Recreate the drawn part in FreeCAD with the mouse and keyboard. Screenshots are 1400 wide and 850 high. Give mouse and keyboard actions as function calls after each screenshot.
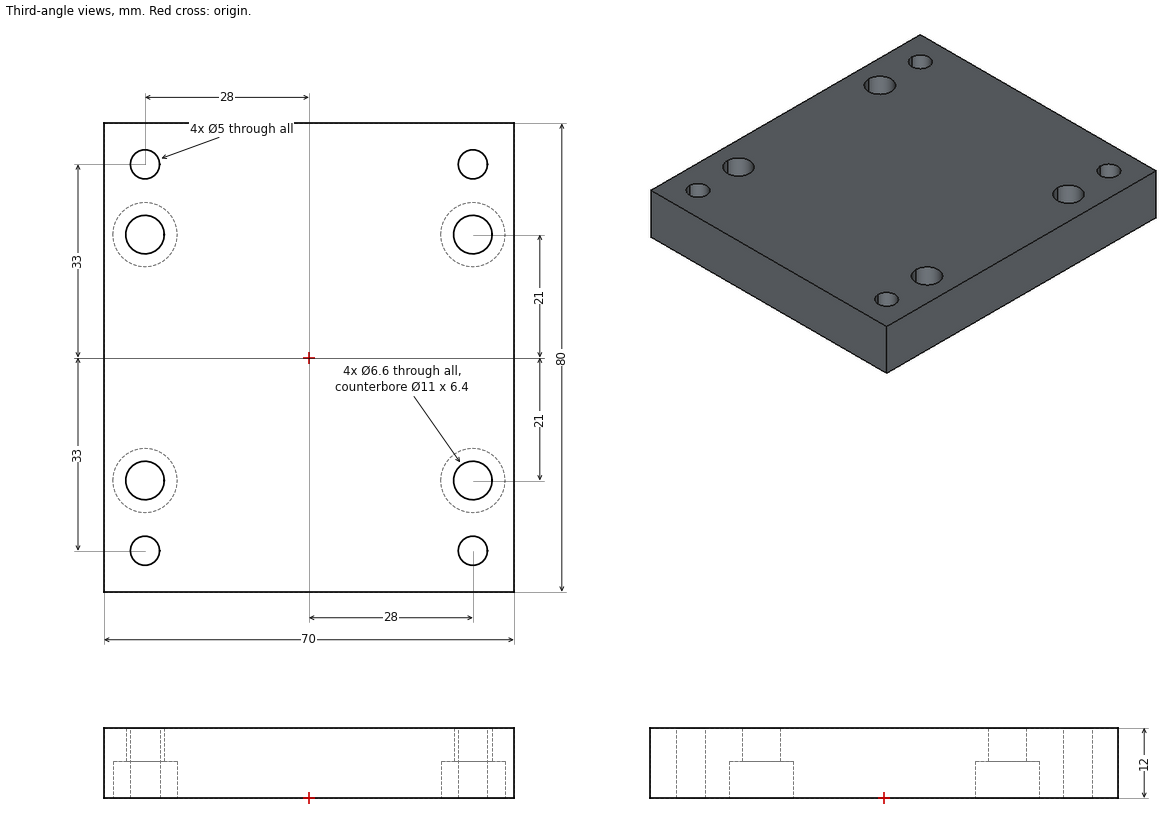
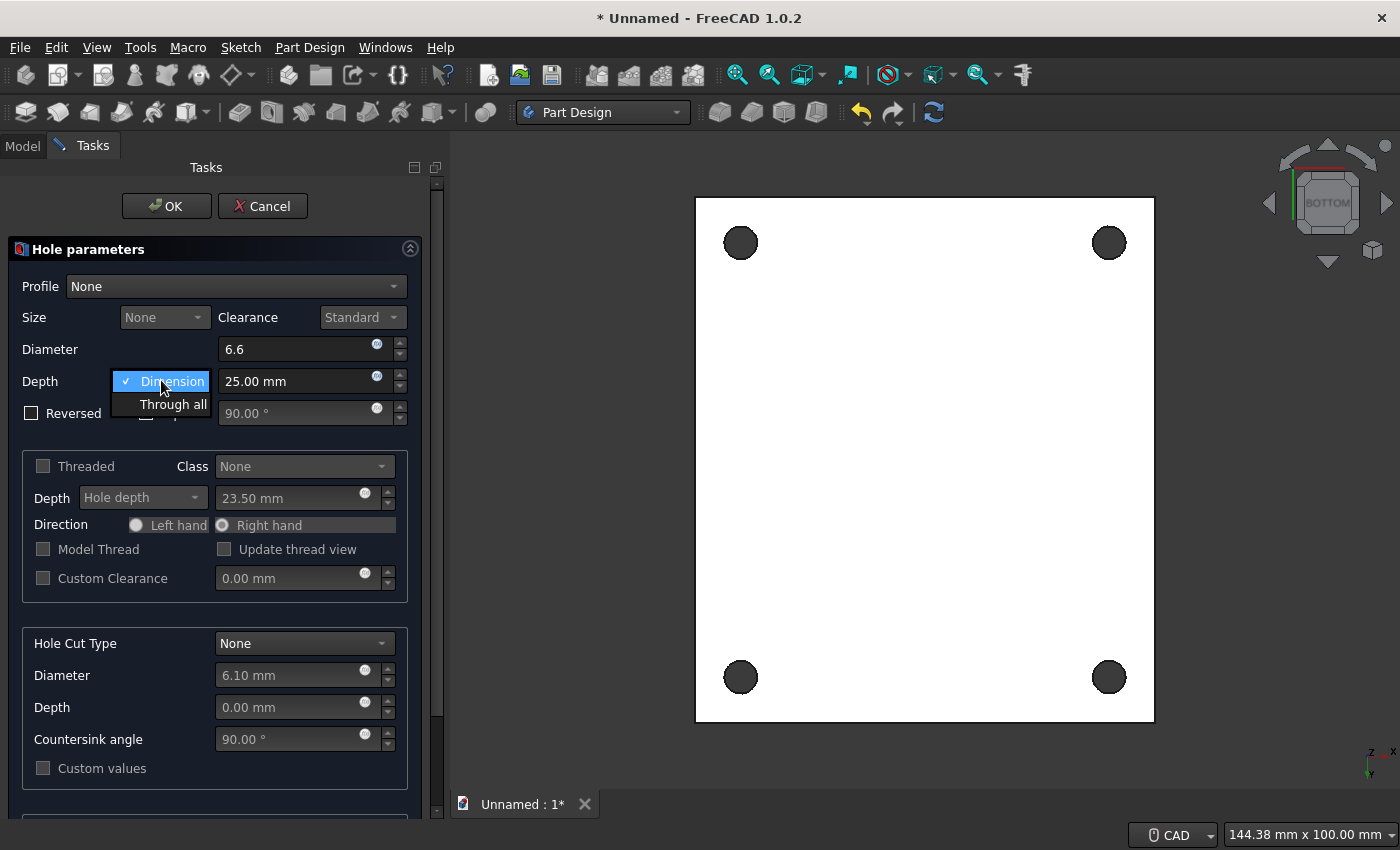
click(160, 404)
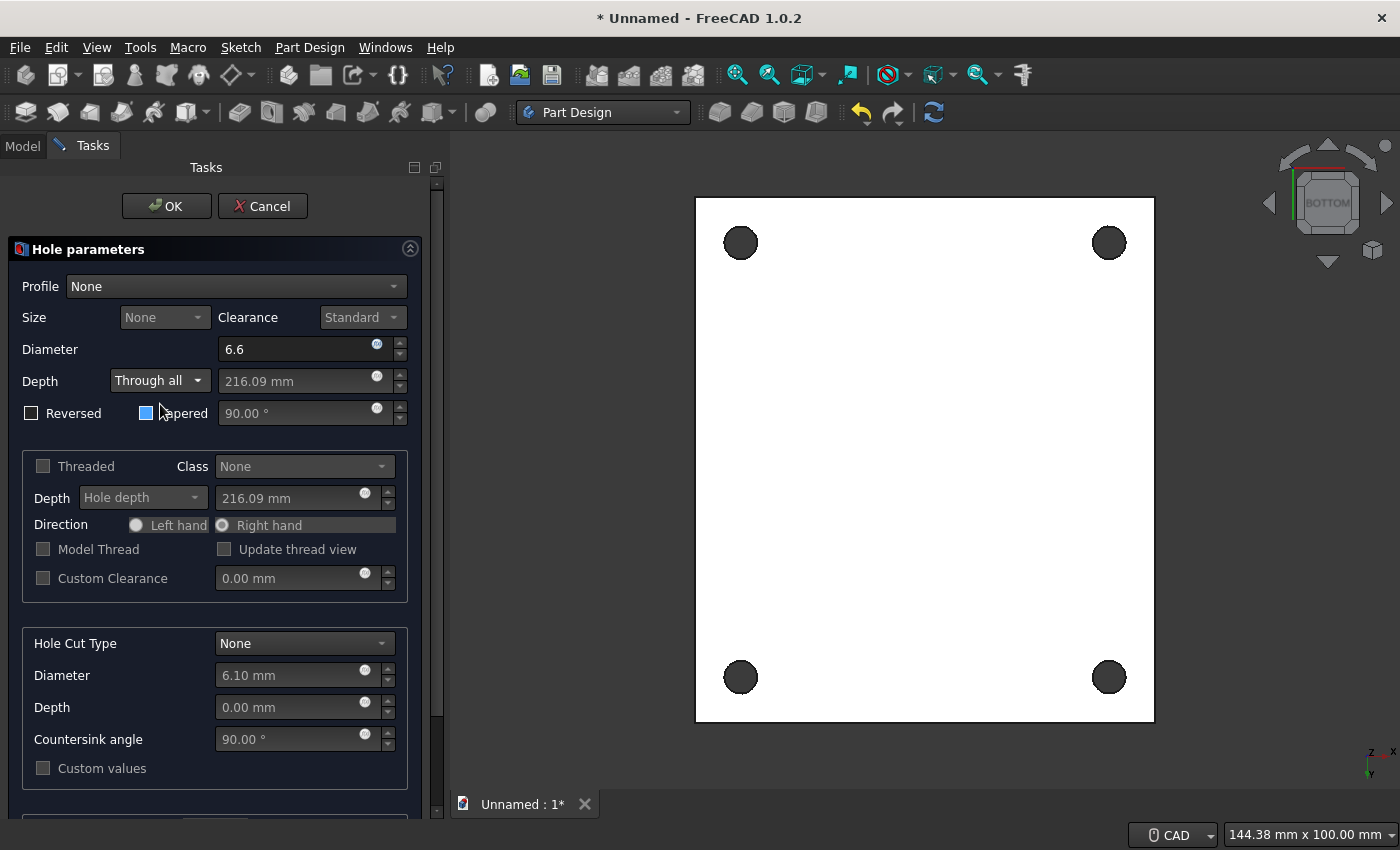
click(30, 413)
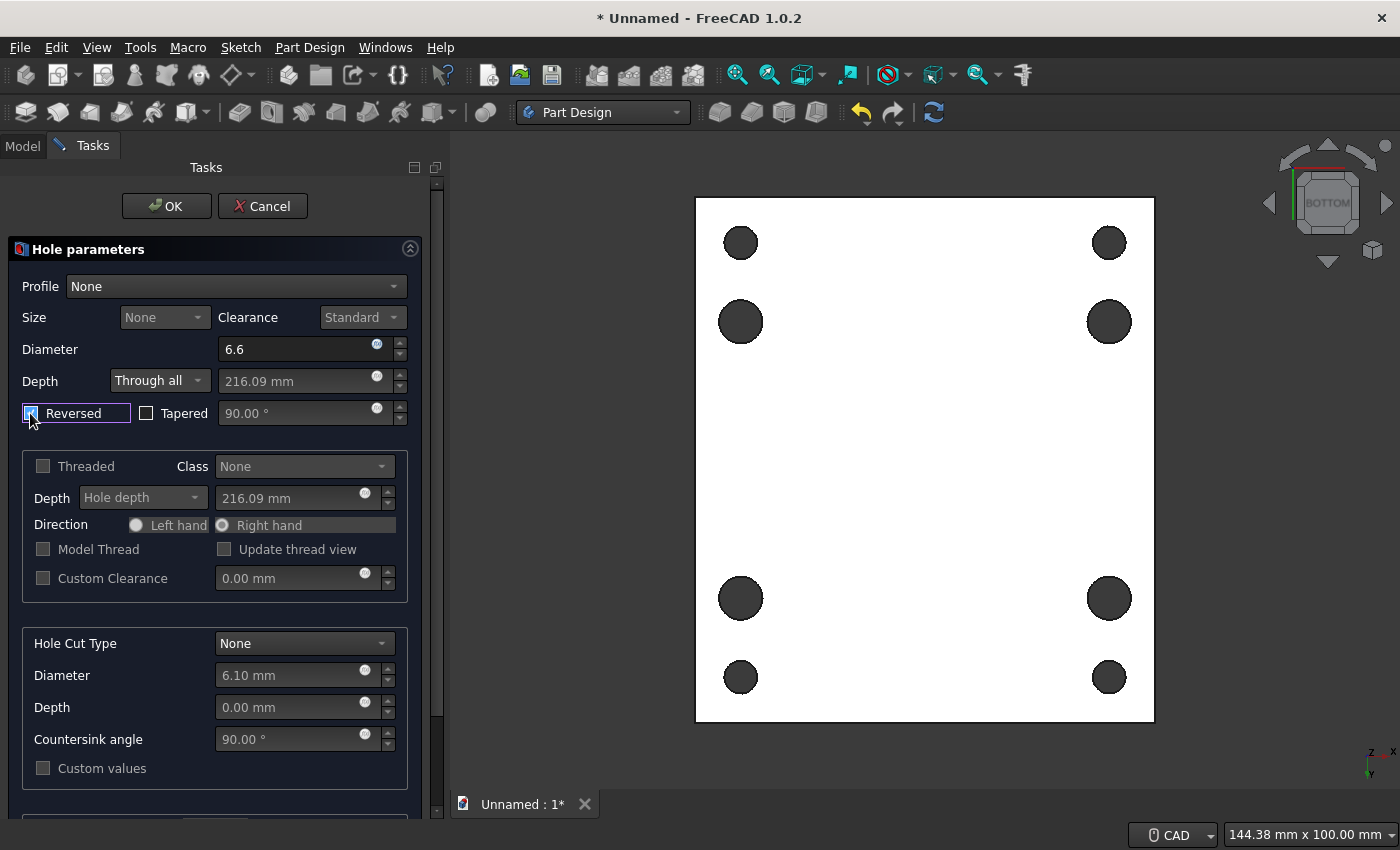
click(306, 644)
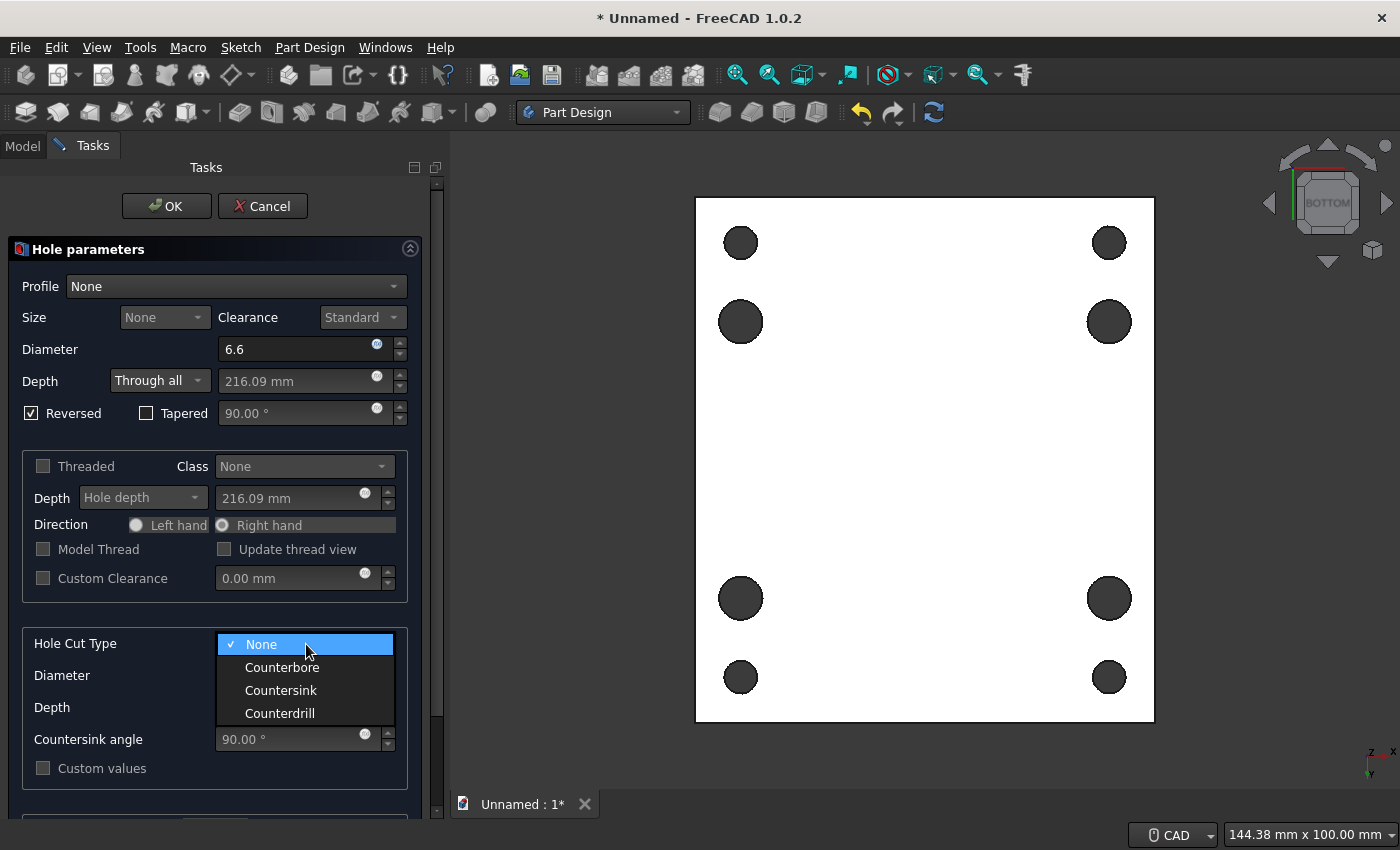
click(304, 668)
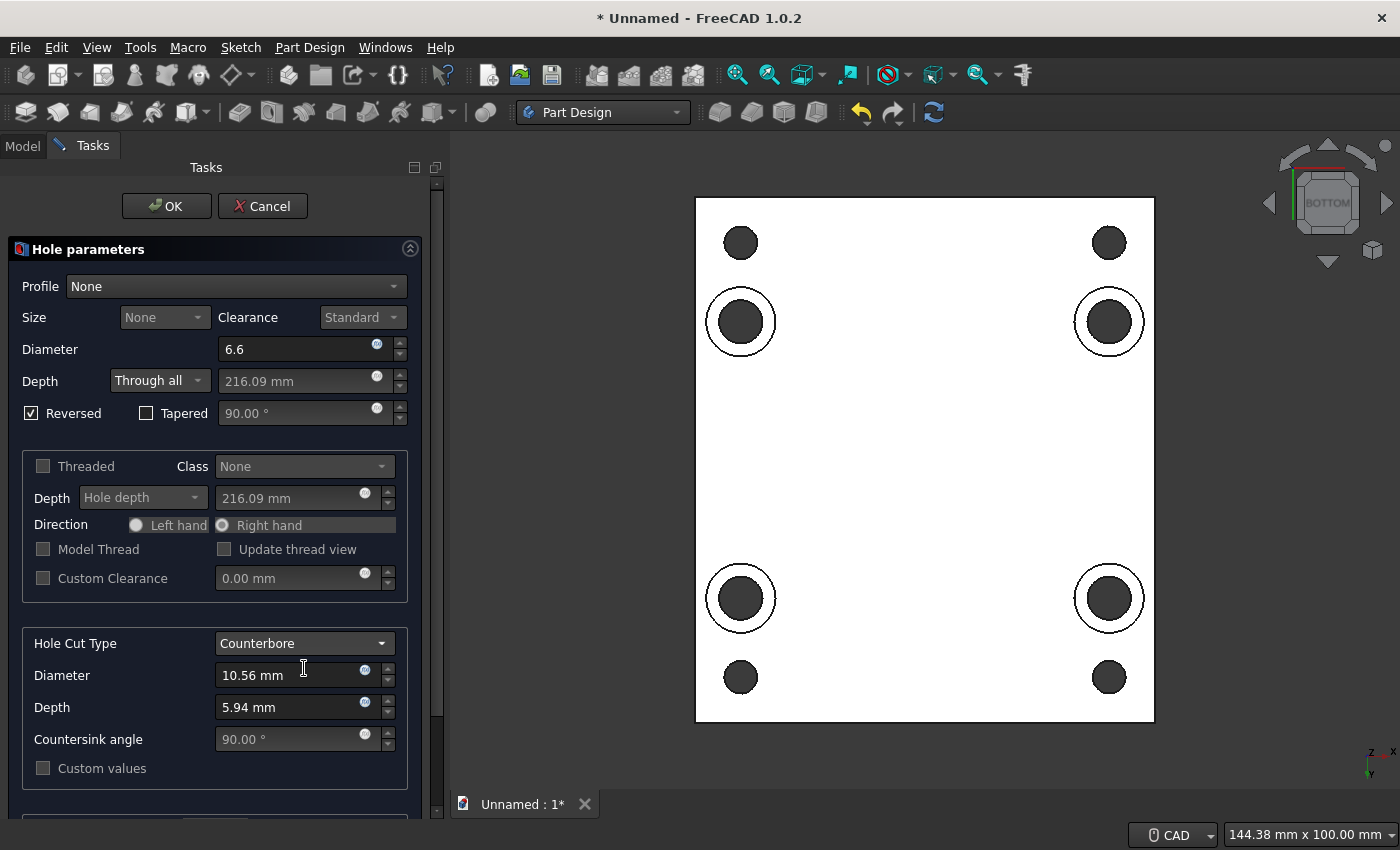
triple_click(298, 675)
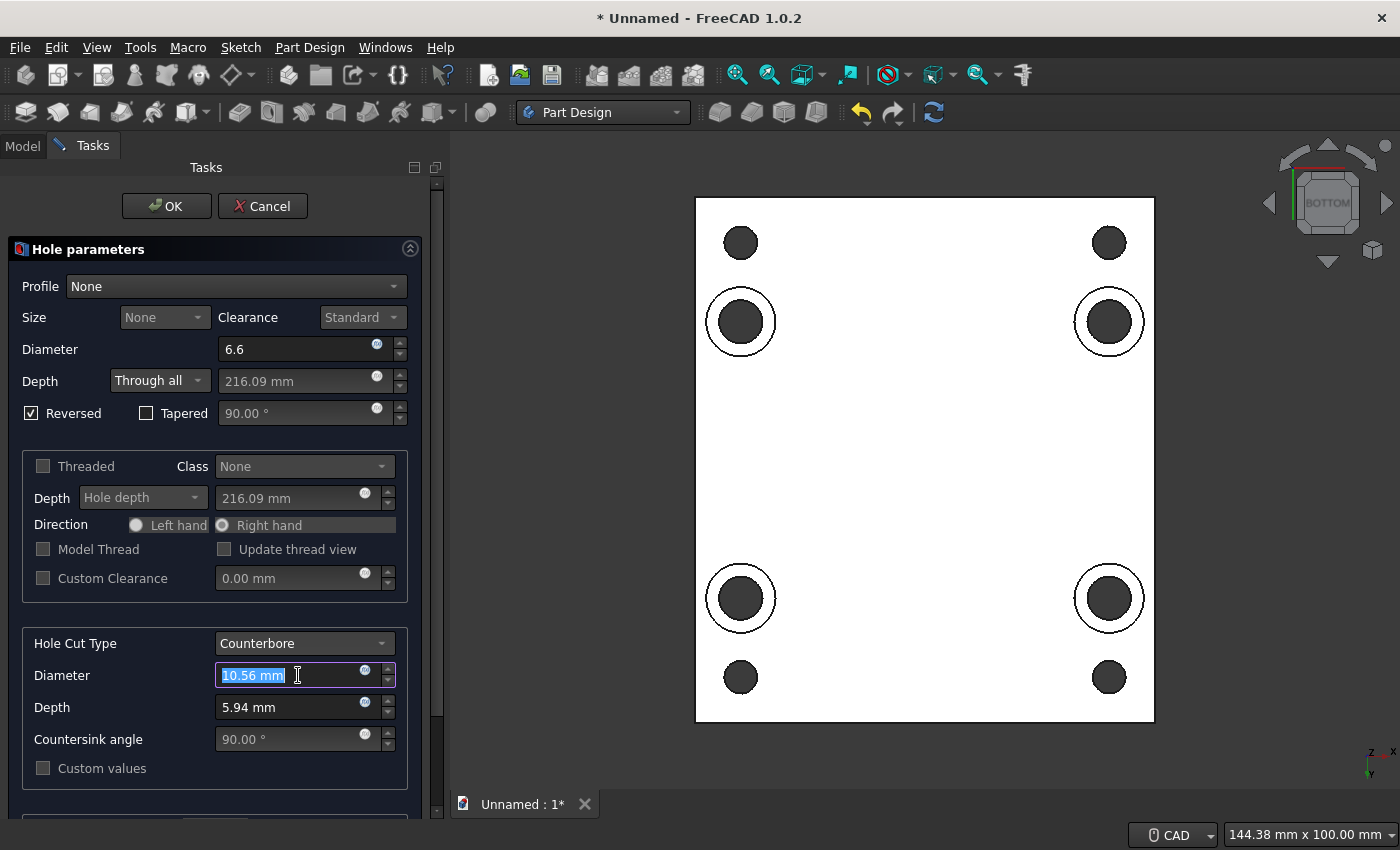
text(11)
key(Tab)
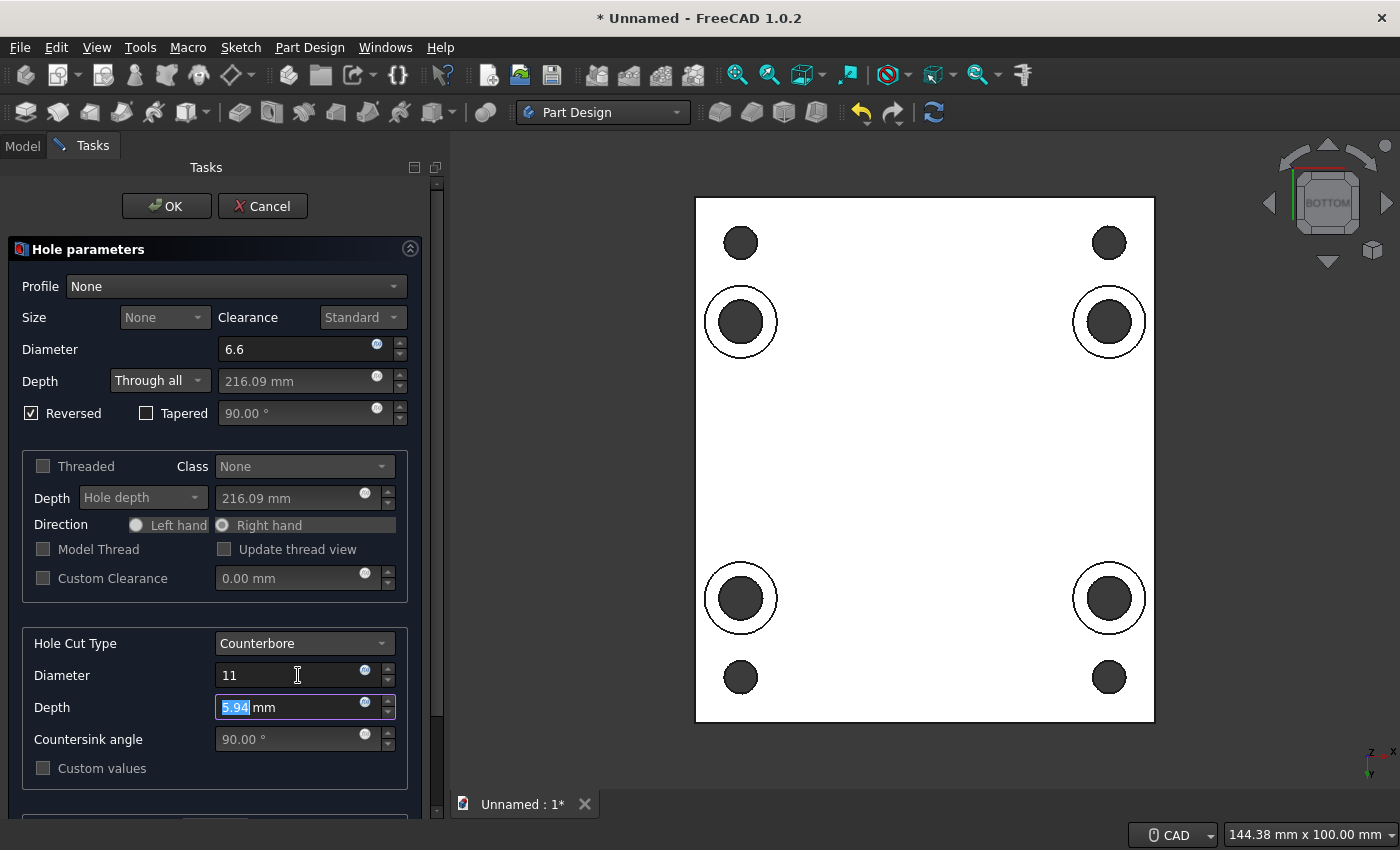
text(6.4)
key(Tab)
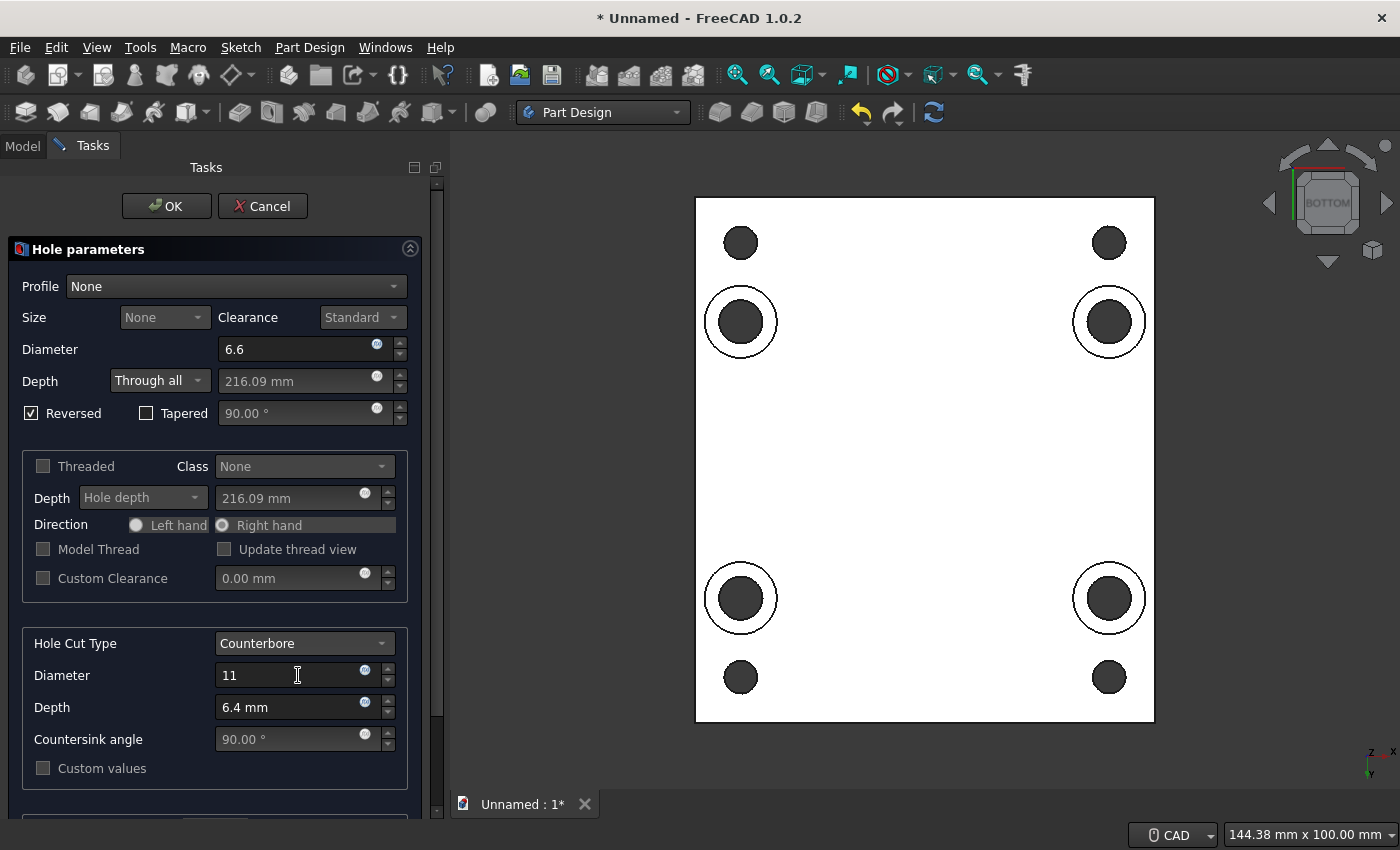
click(167, 206)